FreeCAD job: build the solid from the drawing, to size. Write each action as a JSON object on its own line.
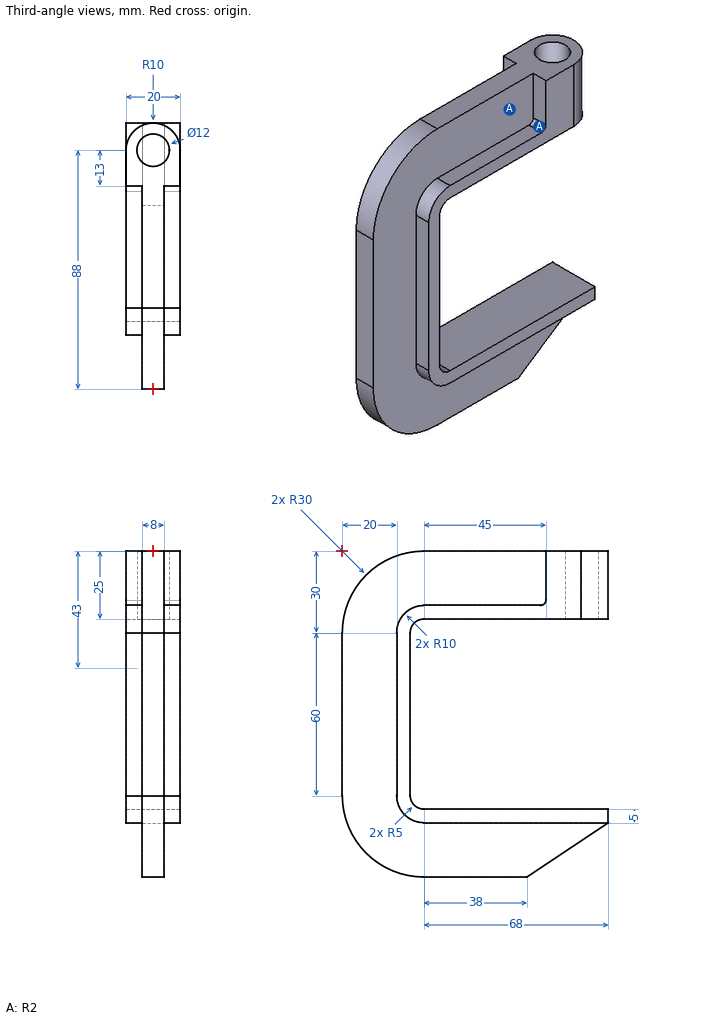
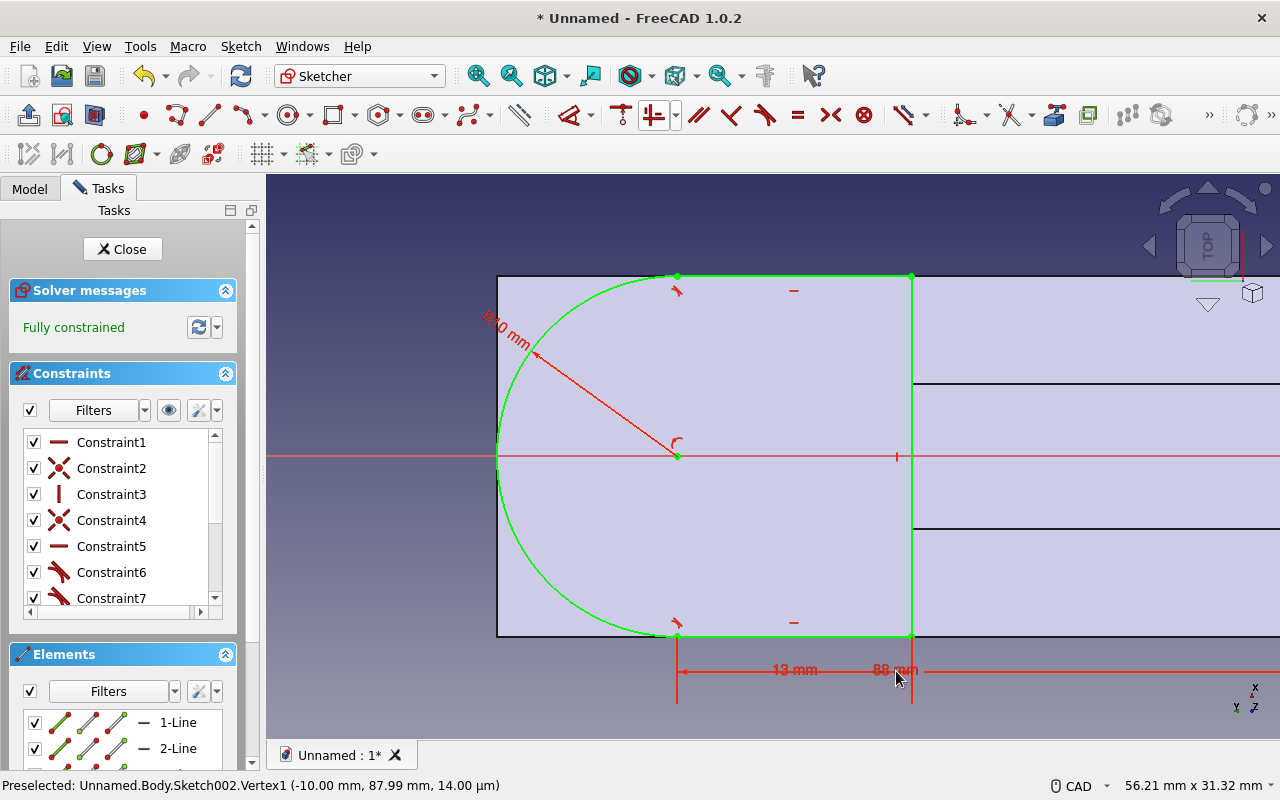
{"action": "left_click", "coordinate": [123, 249]}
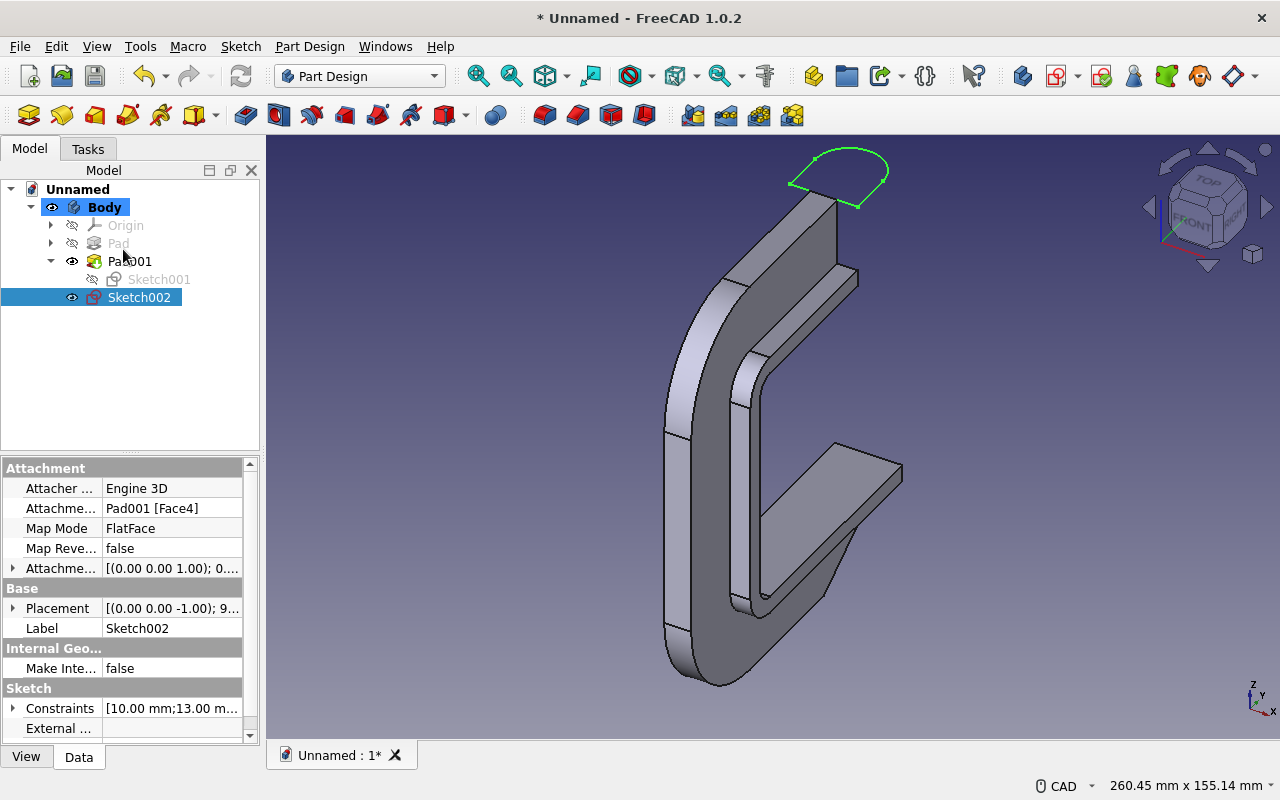
{"action": "left_click", "coordinate": [29, 116]}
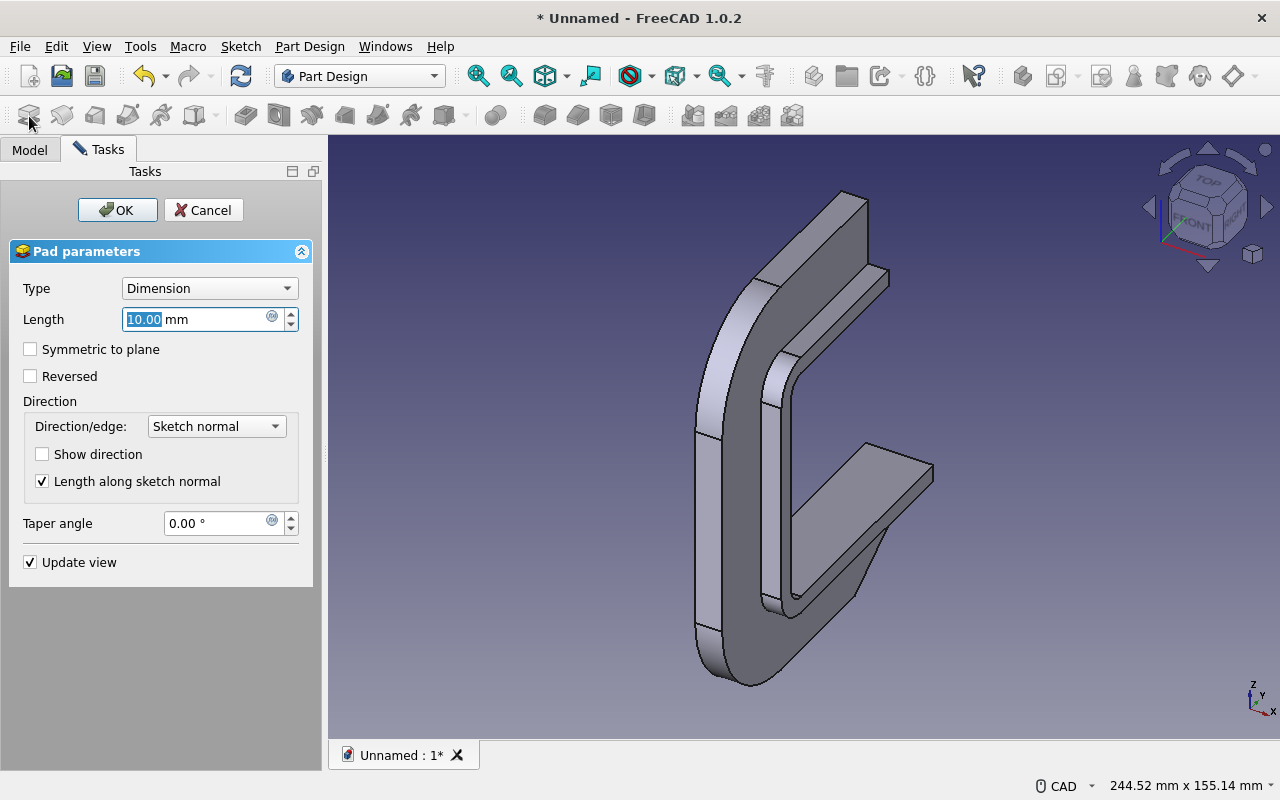
{"action": "type", "text": "25"}
{"action": "key", "text": "Tab"}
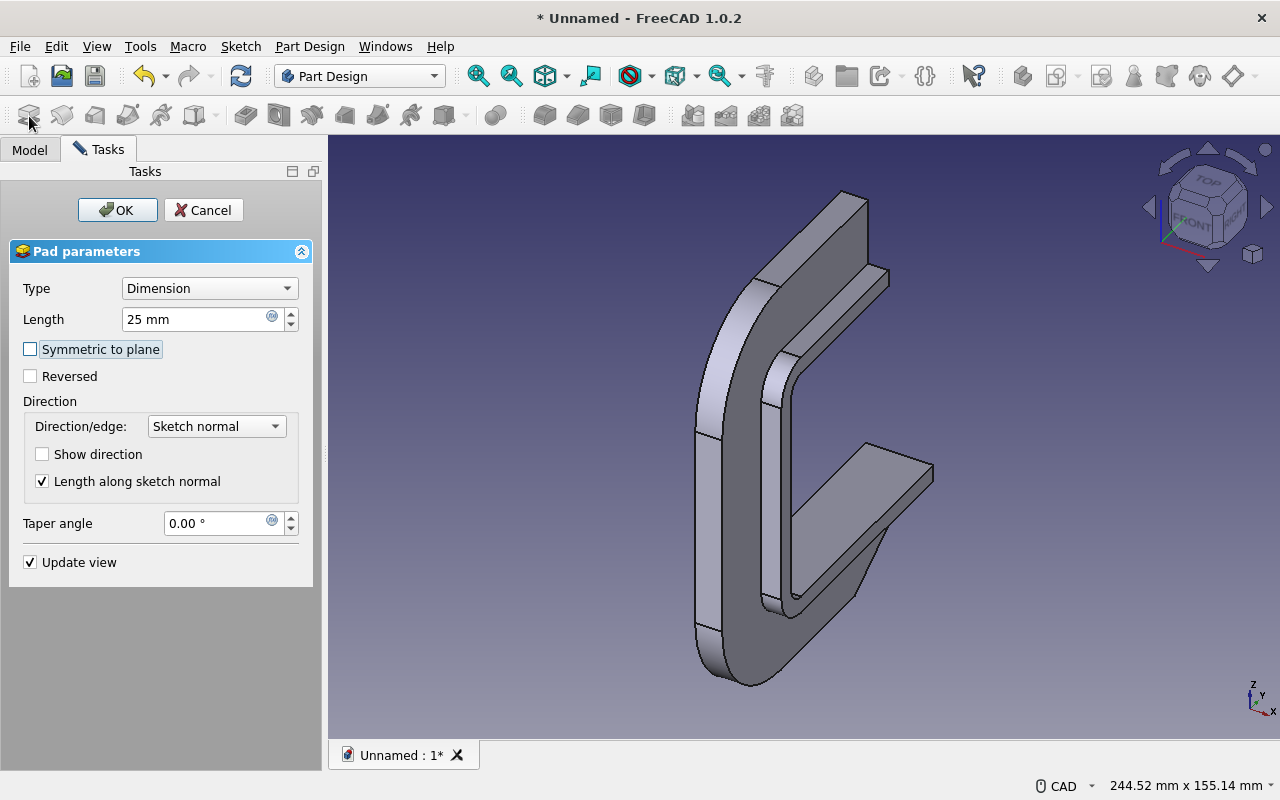
{"action": "left_click", "coordinate": [31, 376]}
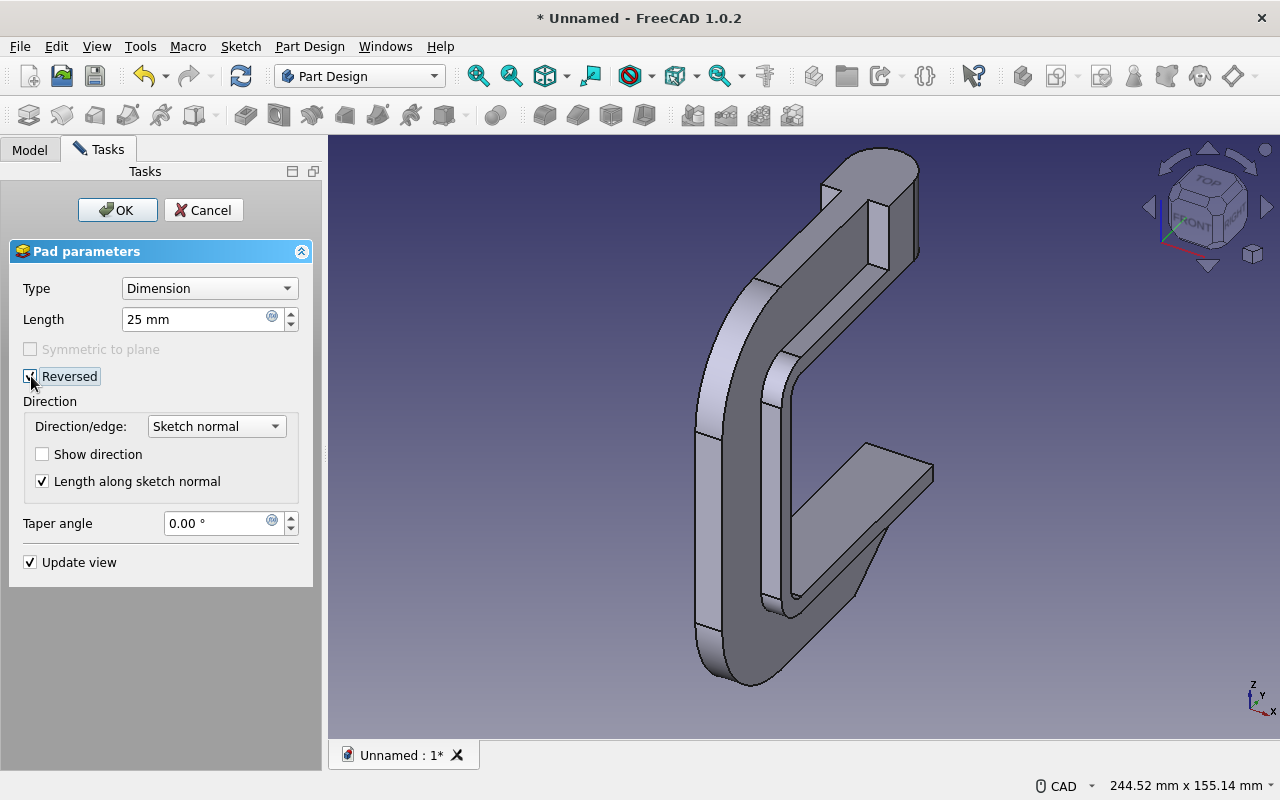
{"action": "left_click", "coordinate": [118, 210]}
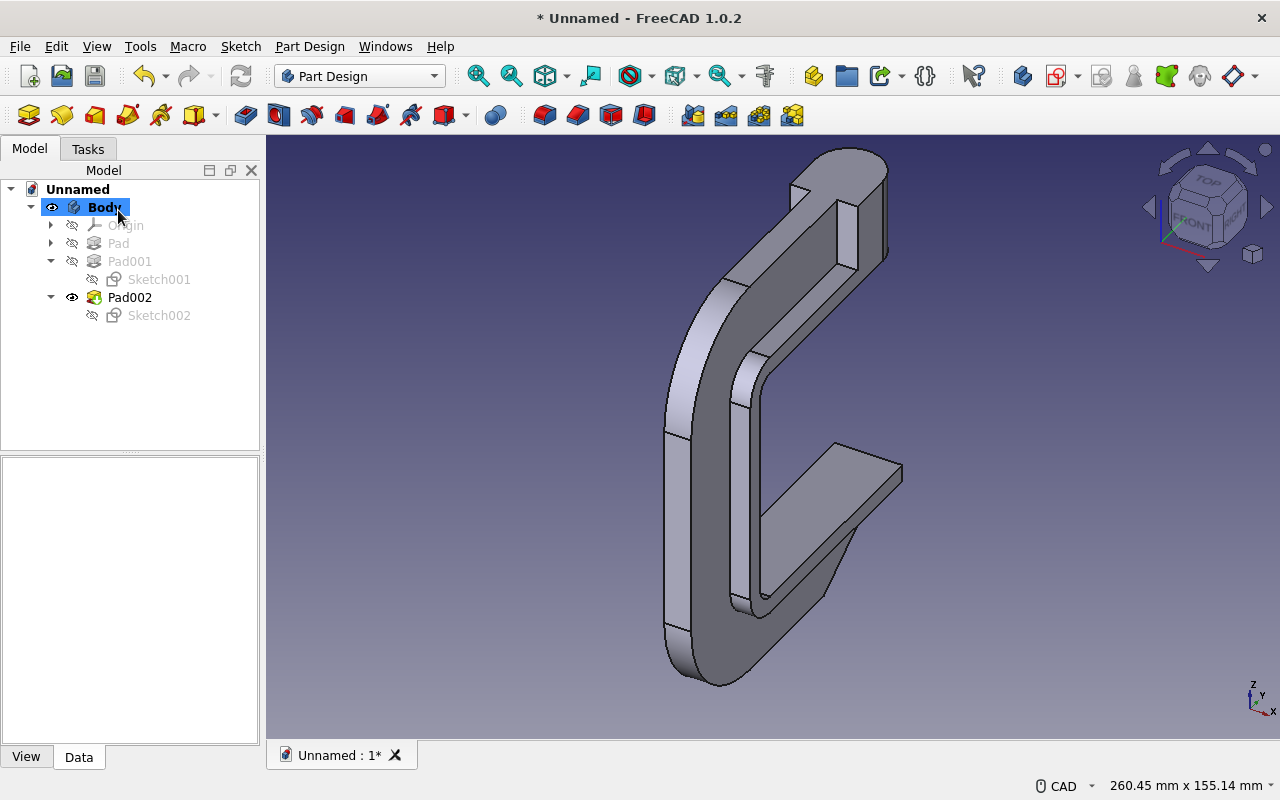
{"action": "left_click", "coordinate": [840, 178]}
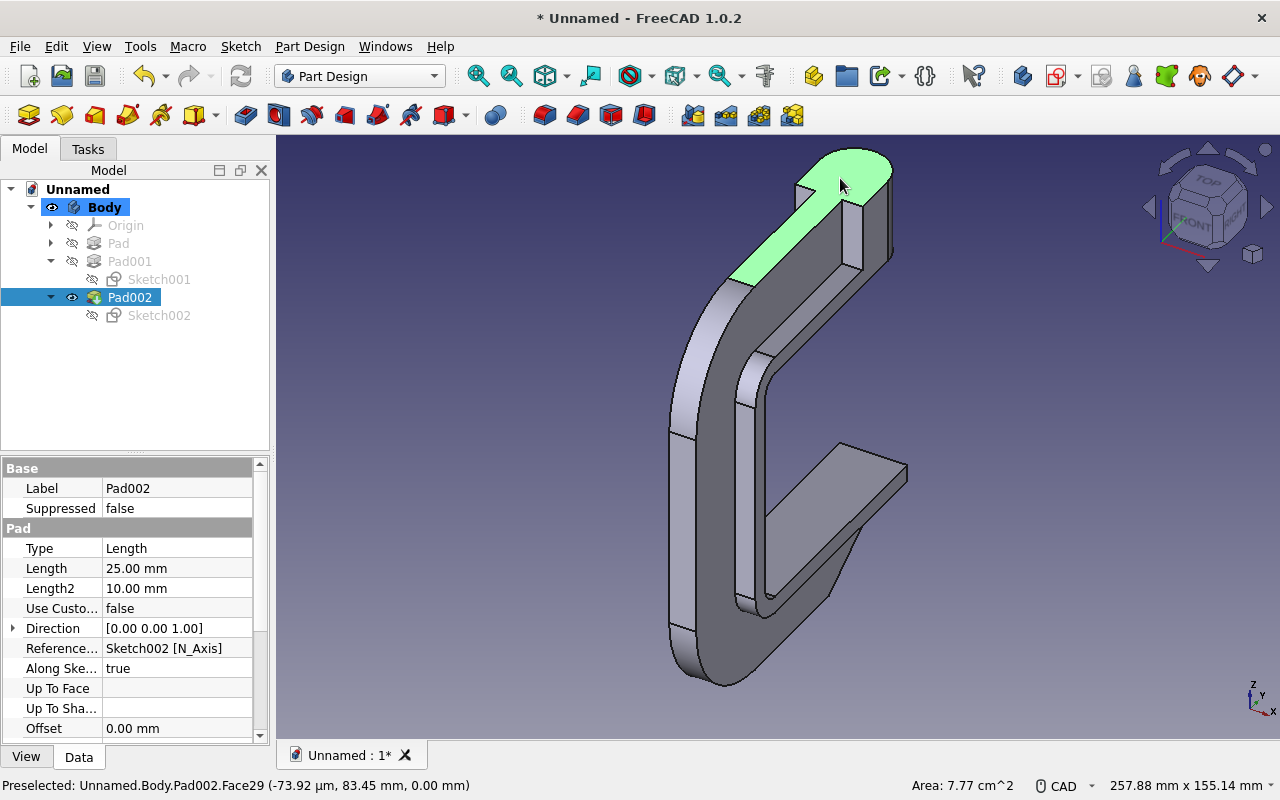
{"action": "left_click", "coordinate": [1056, 76]}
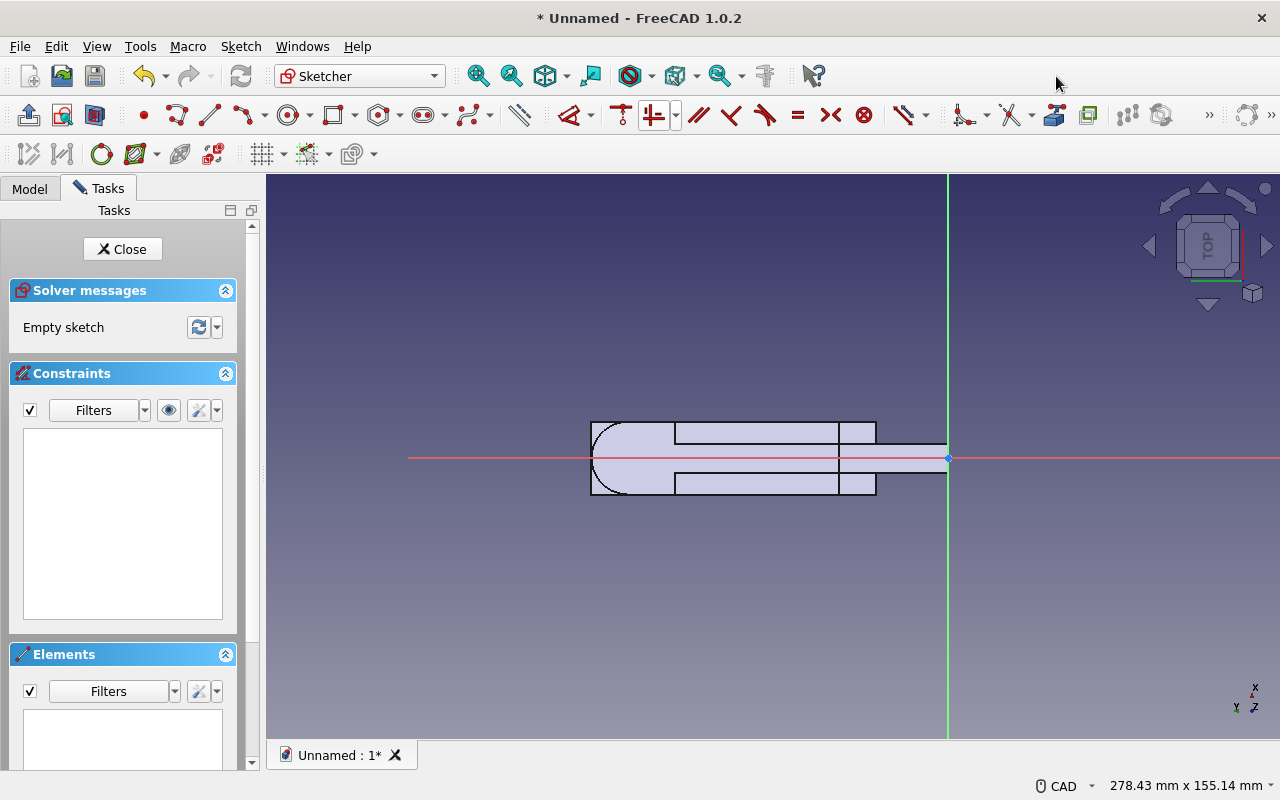
{"action": "scroll", "coordinate": [618, 458], "scroll_direction": "up", "scroll_amount": 11}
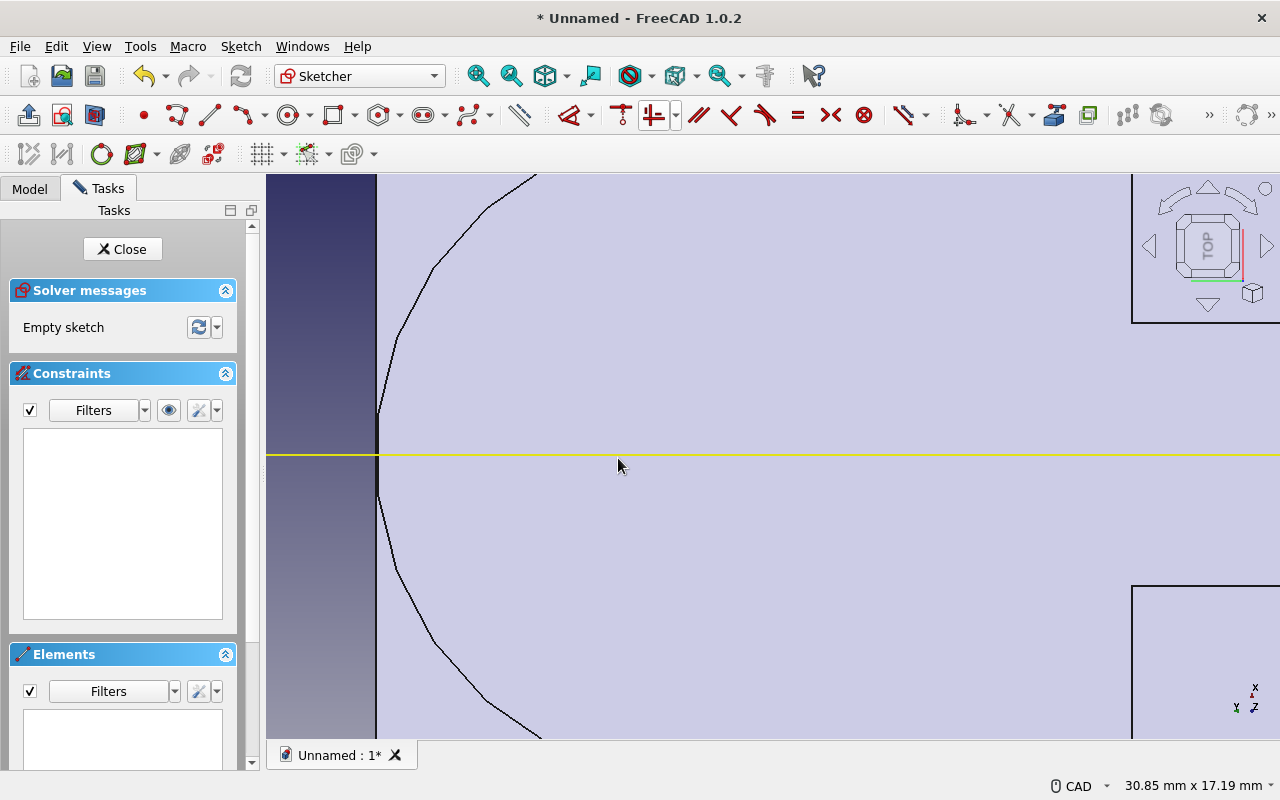
{"action": "key", "text": "g c"}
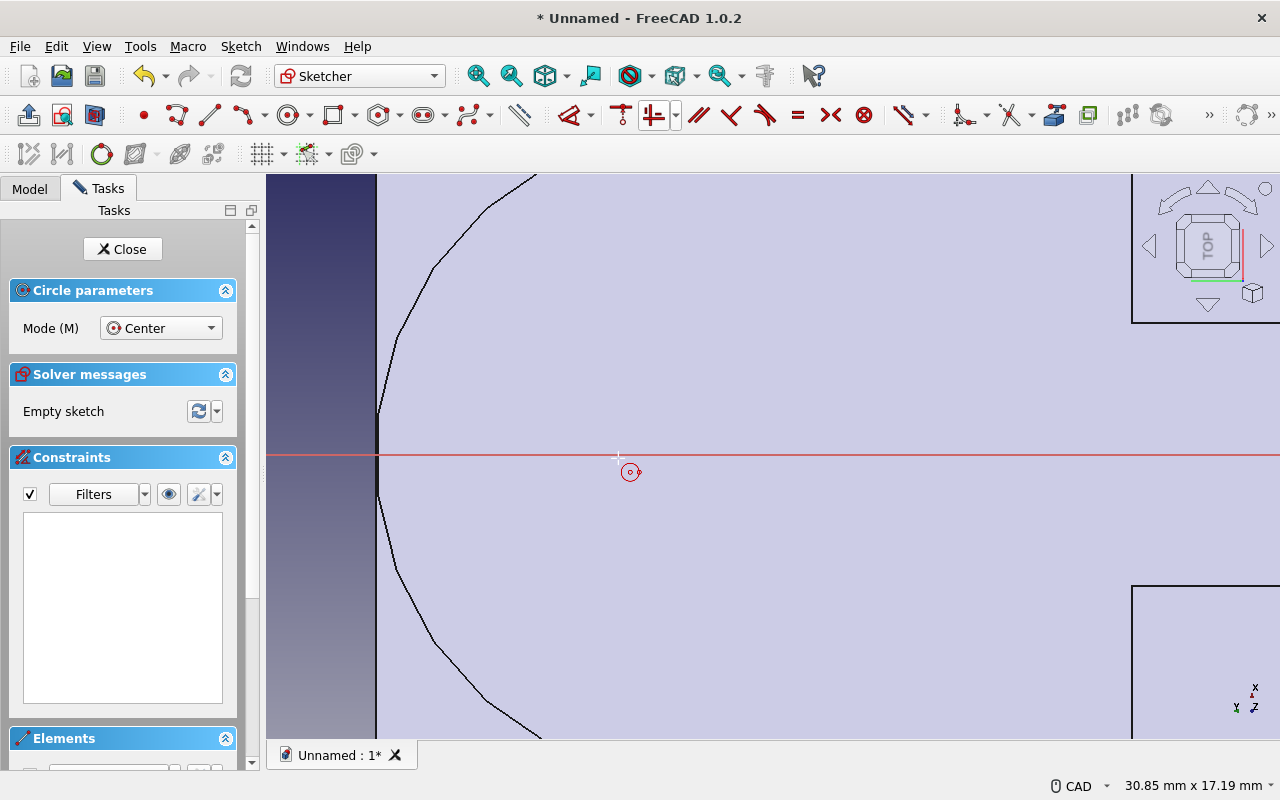
{"action": "left_click", "coordinate": [704, 455]}
{"action": "mouse_move", "coordinate": [844, 315]}